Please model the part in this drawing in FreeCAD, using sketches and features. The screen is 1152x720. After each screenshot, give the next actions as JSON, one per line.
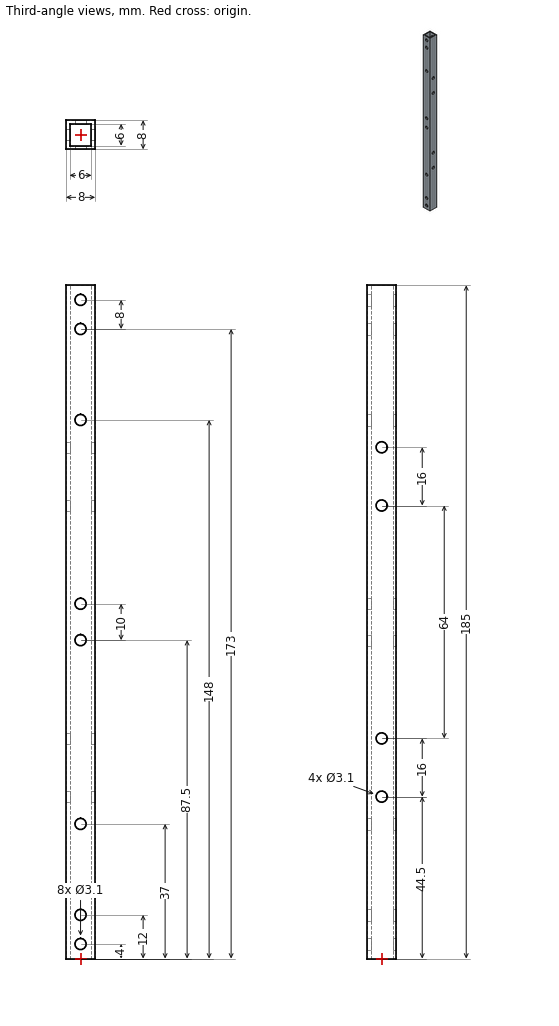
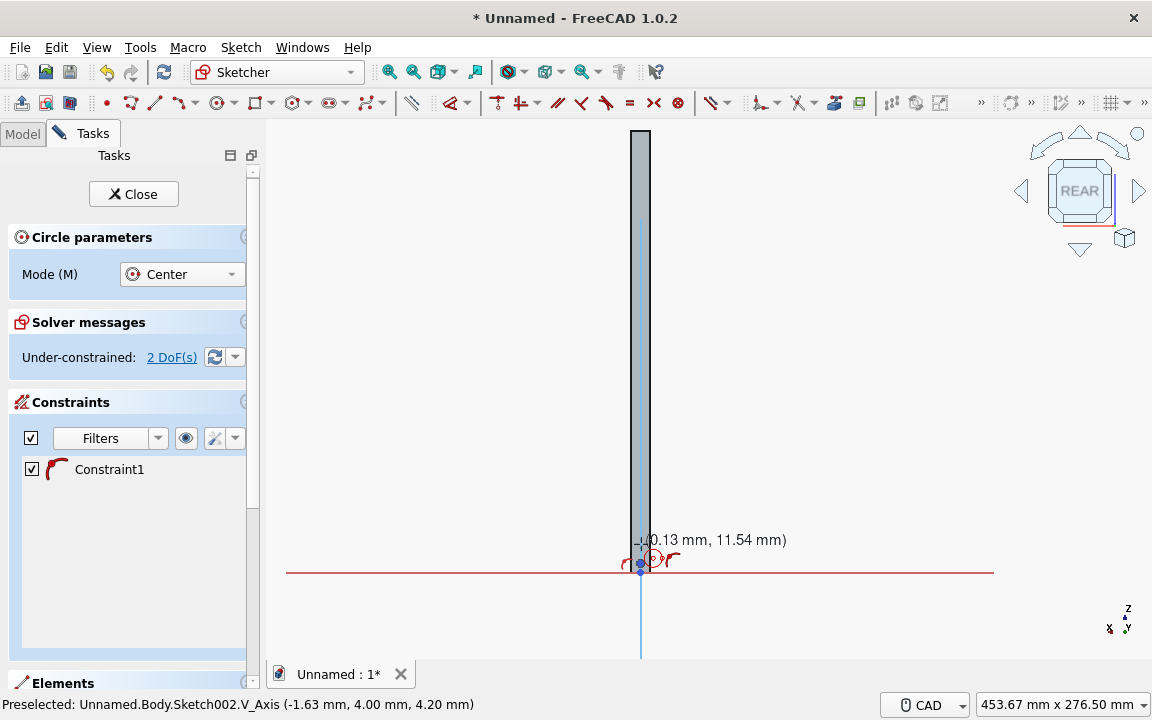
{"action": "left_click", "coordinate": [640, 544]}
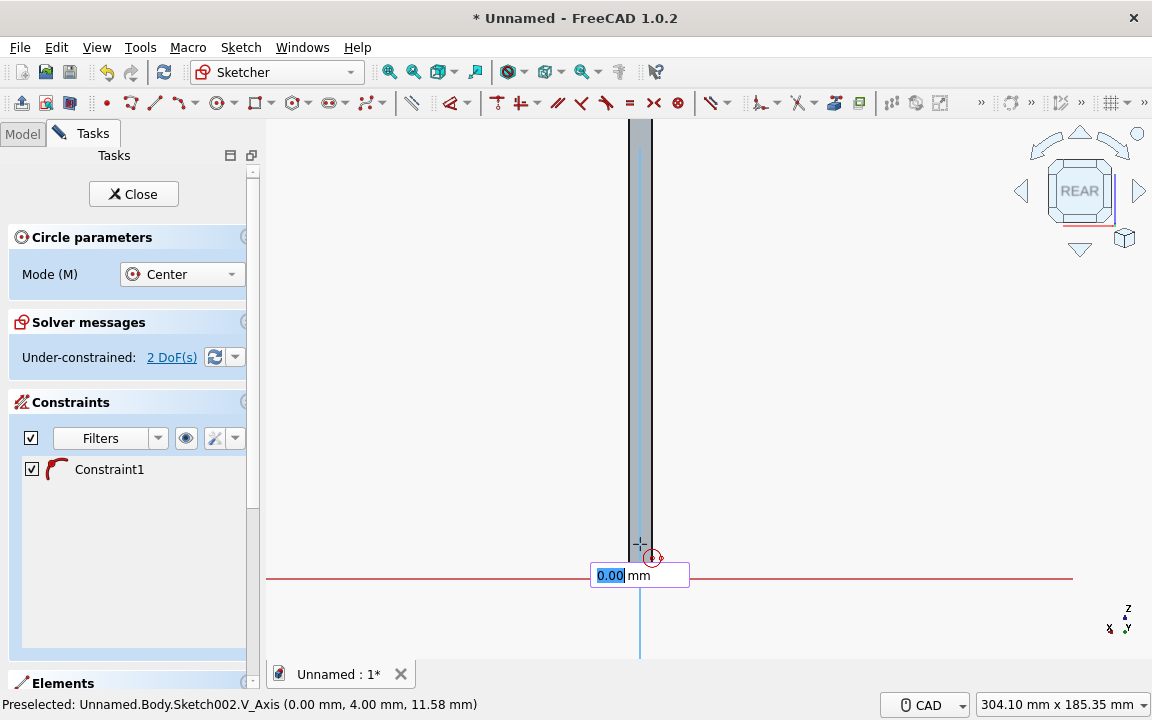
{"action": "scroll", "coordinate": [645, 542], "scroll_direction": "up", "scroll_amount": 7}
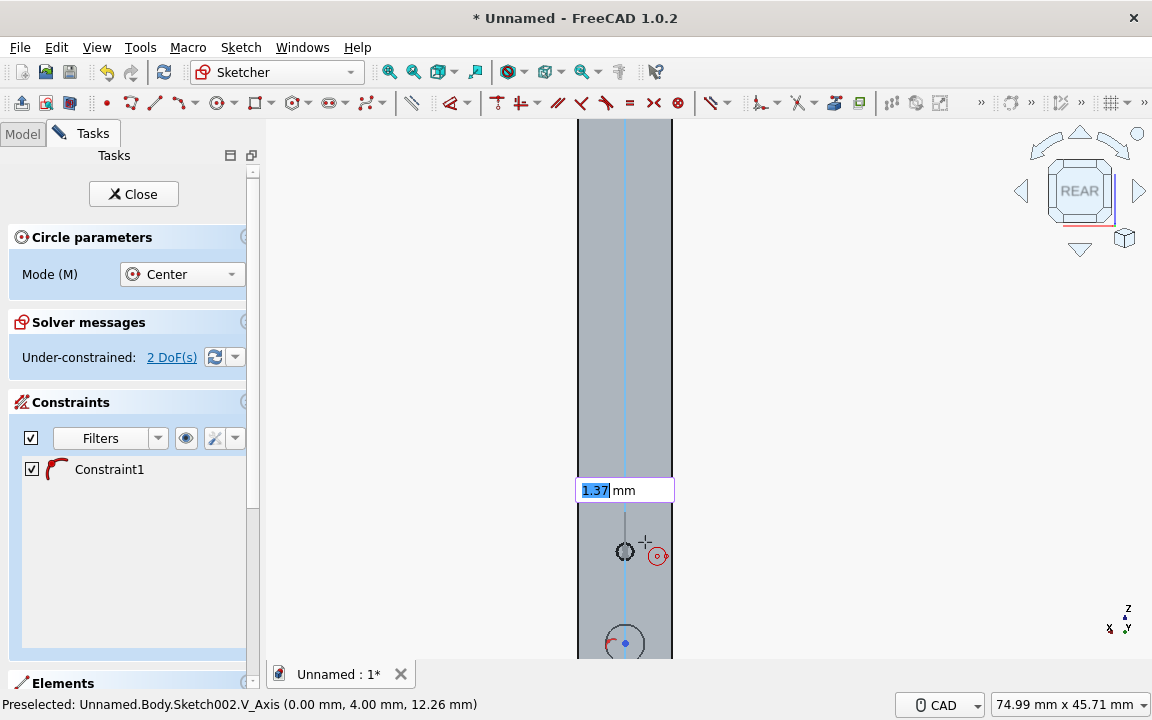
{"action": "left_click", "coordinate": [642, 540]}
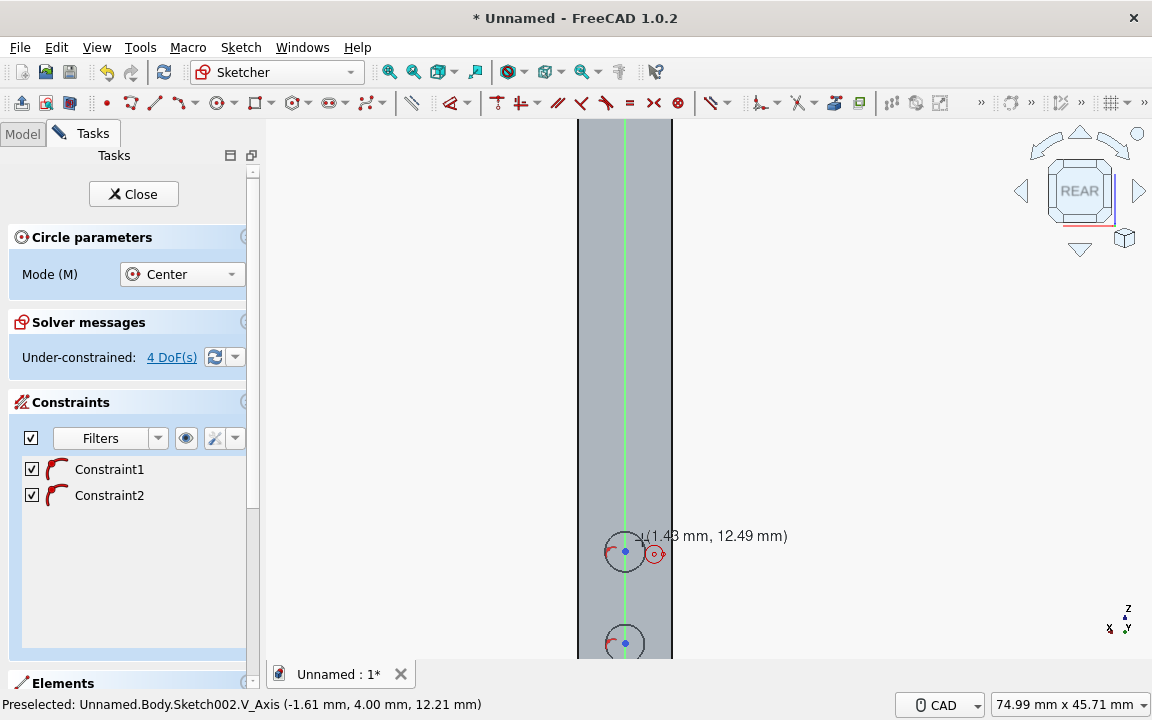
{"action": "scroll", "coordinate": [644, 543], "scroll_direction": "down", "scroll_amount": 9}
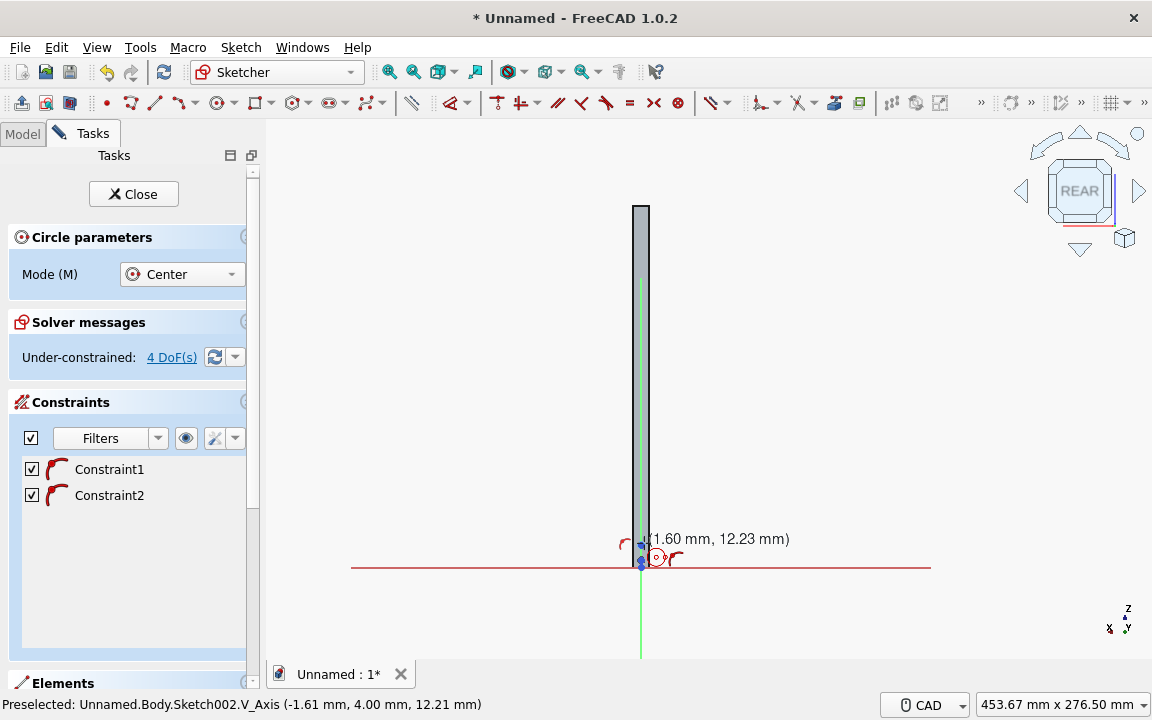
{"action": "scroll", "coordinate": [641, 230], "scroll_direction": "up", "scroll_amount": 11}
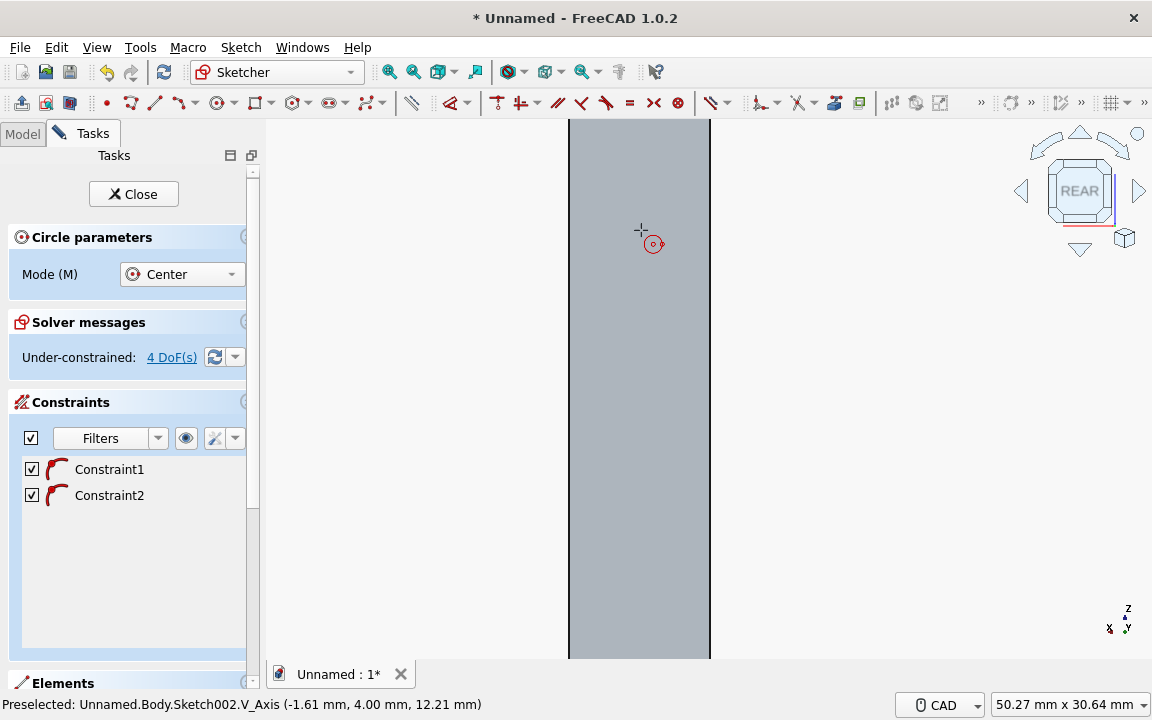
{"action": "scroll", "coordinate": [641, 230], "scroll_direction": "down", "scroll_amount": 11}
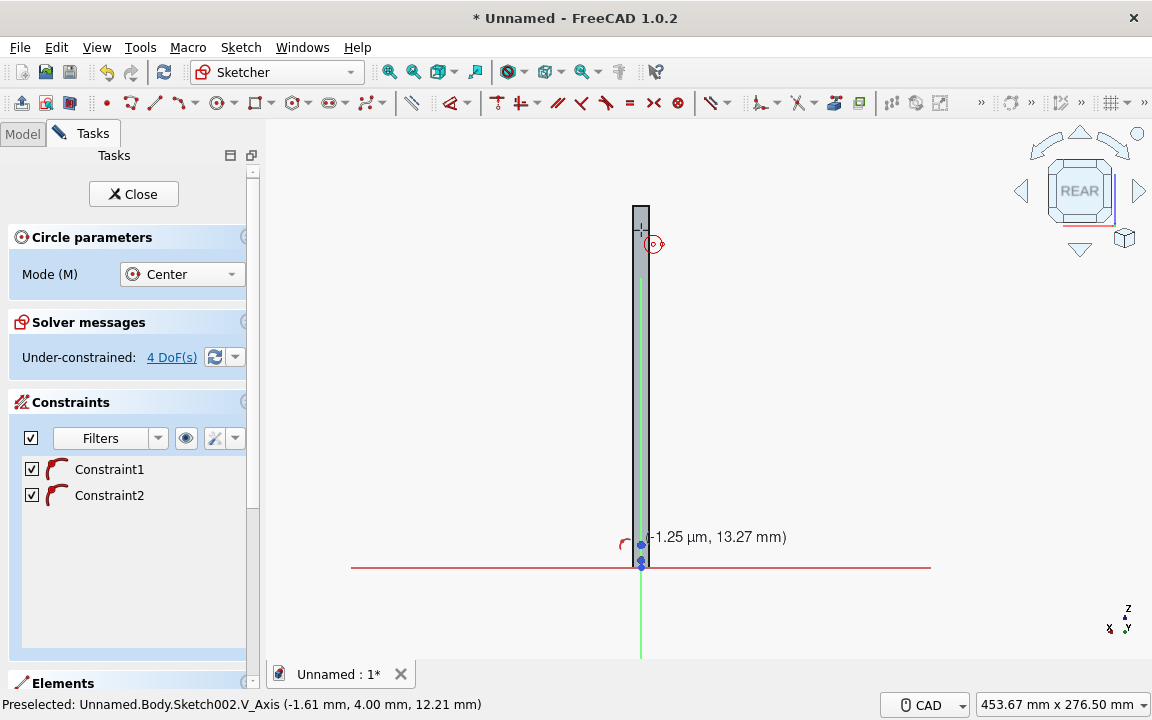
{"action": "left_click", "coordinate": [641, 230]}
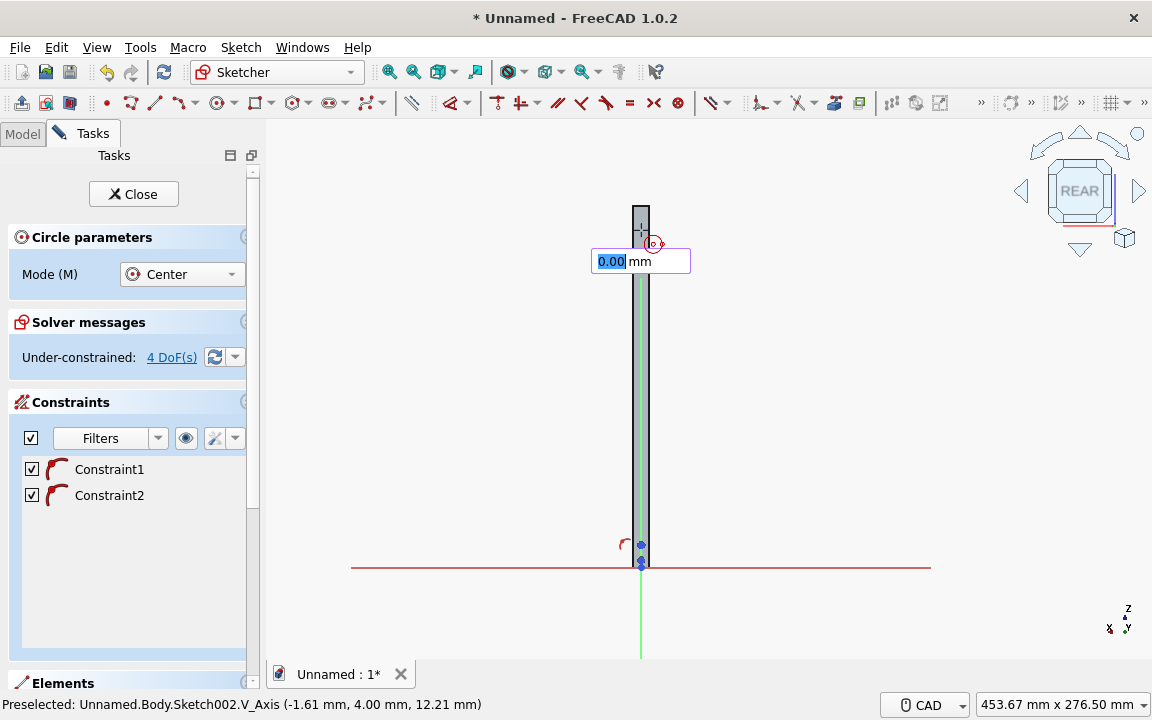
{"action": "scroll", "coordinate": [644, 229], "scroll_direction": "up", "scroll_amount": 9}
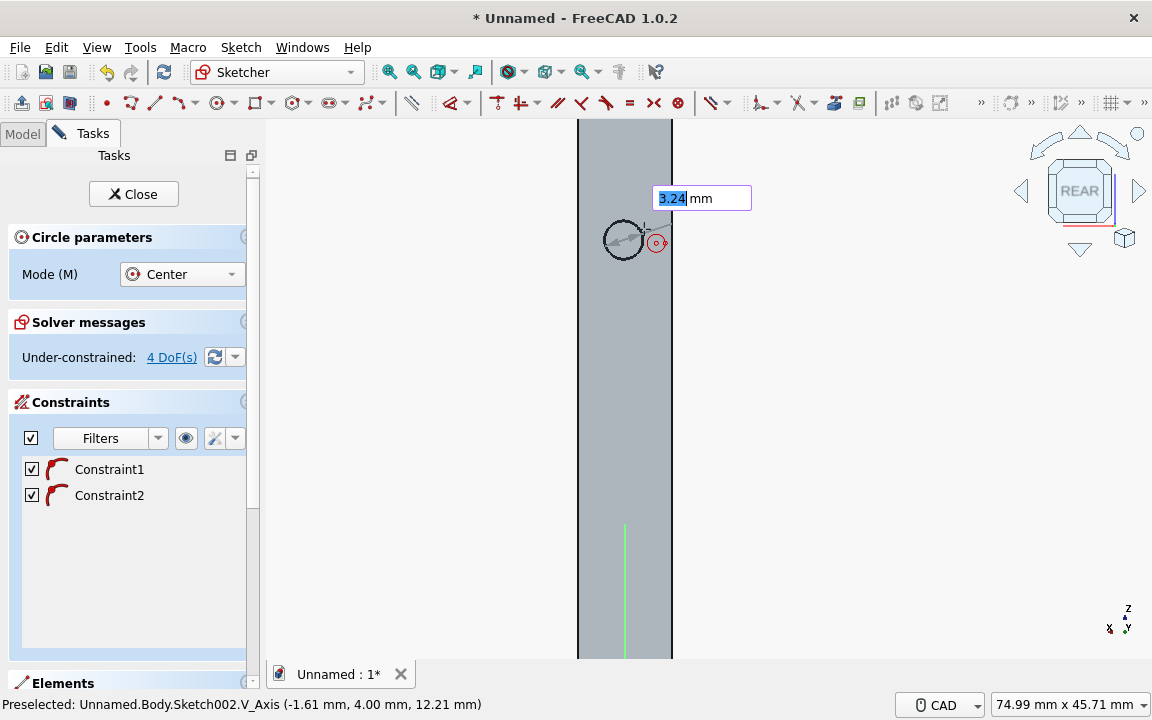
{"action": "left_click", "coordinate": [642, 227]}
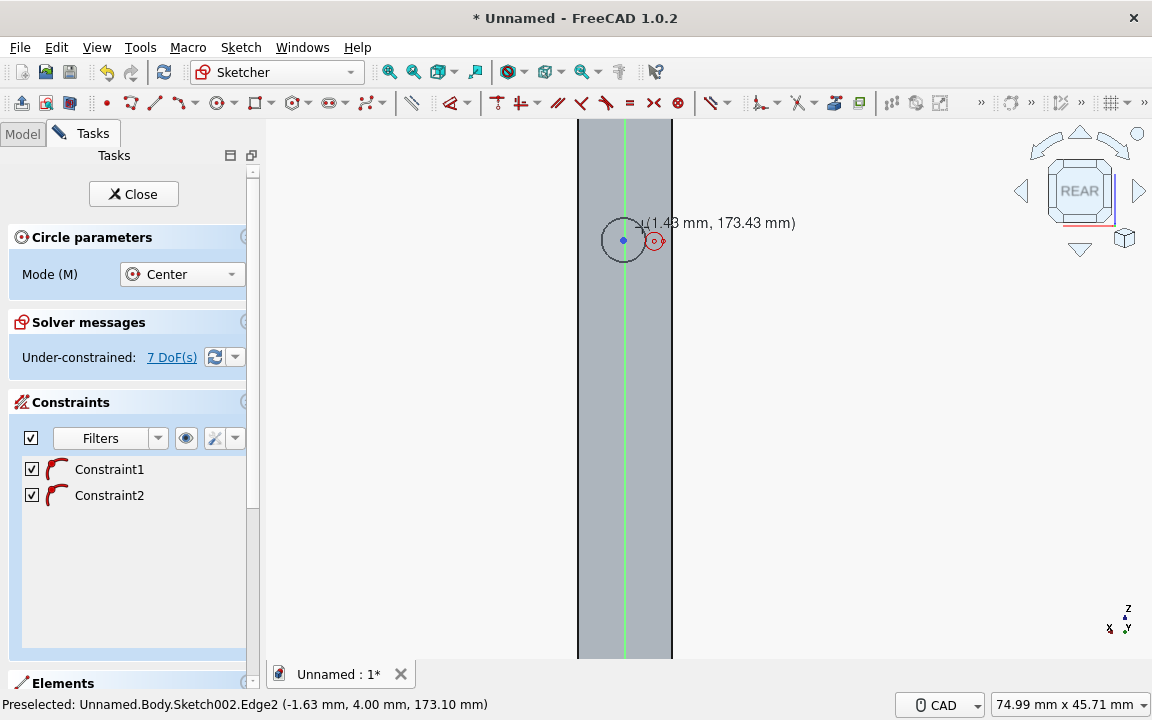
{"action": "scroll", "coordinate": [644, 229], "scroll_direction": "down", "scroll_amount": 9}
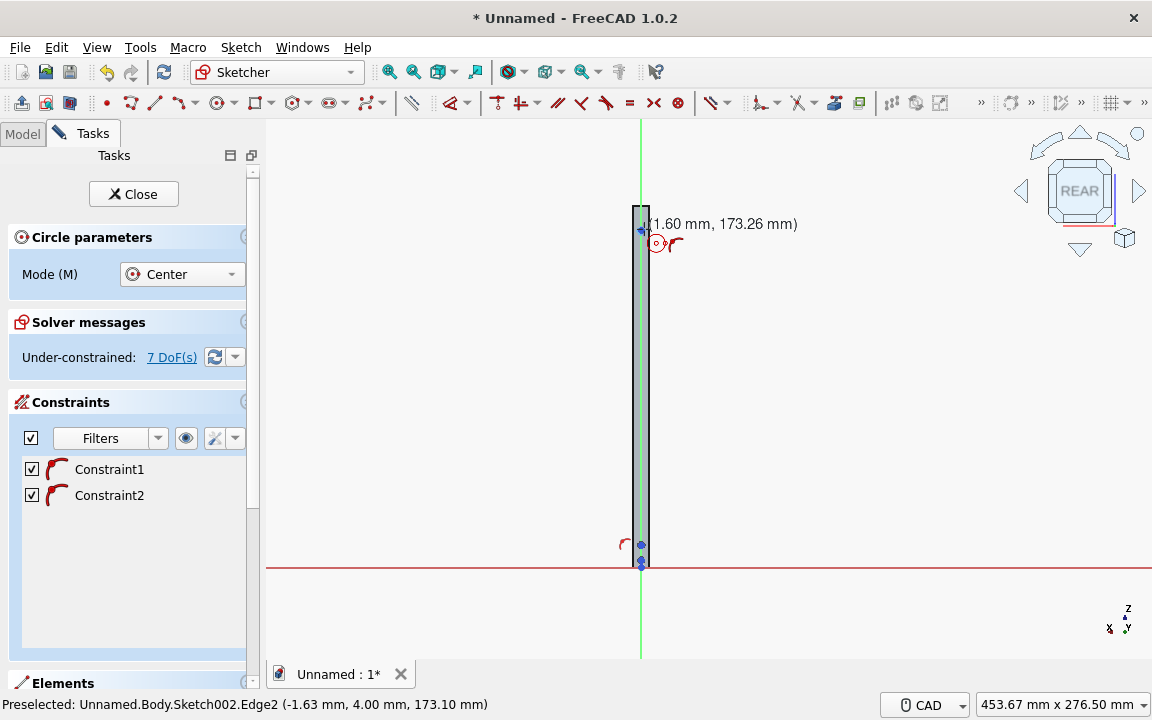
{"action": "scroll", "coordinate": [641, 214], "scroll_direction": "up", "scroll_amount": 11}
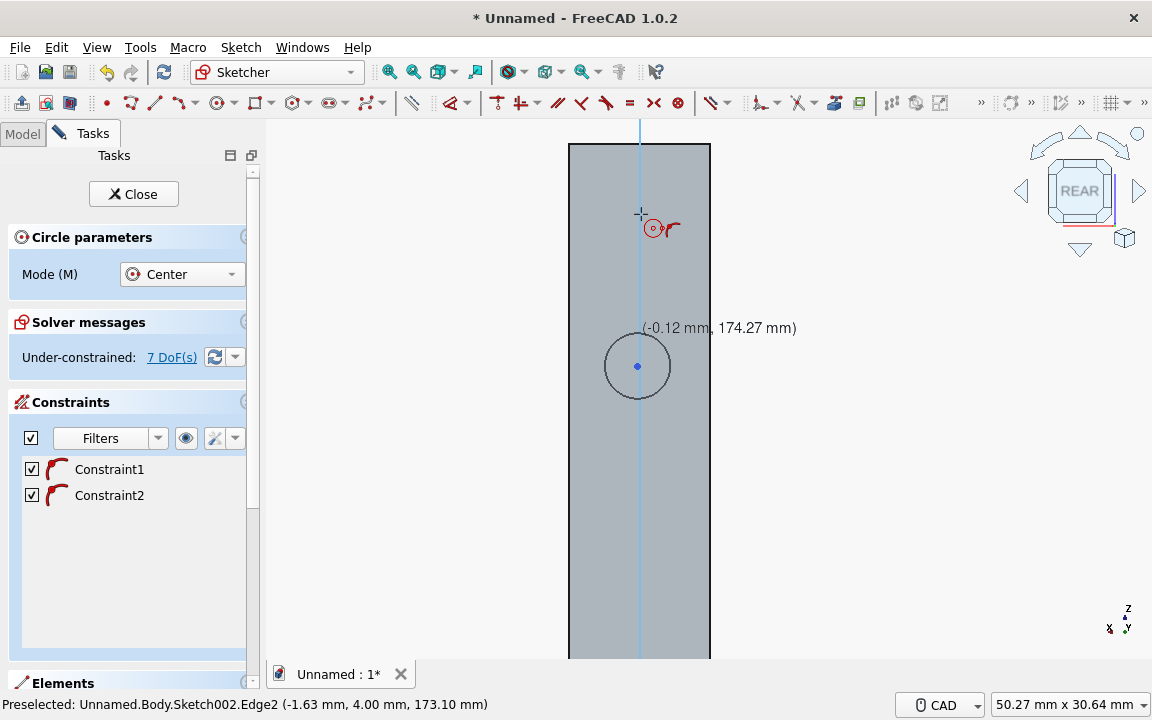
{"action": "scroll", "coordinate": [641, 214], "scroll_direction": "down", "scroll_amount": 11}